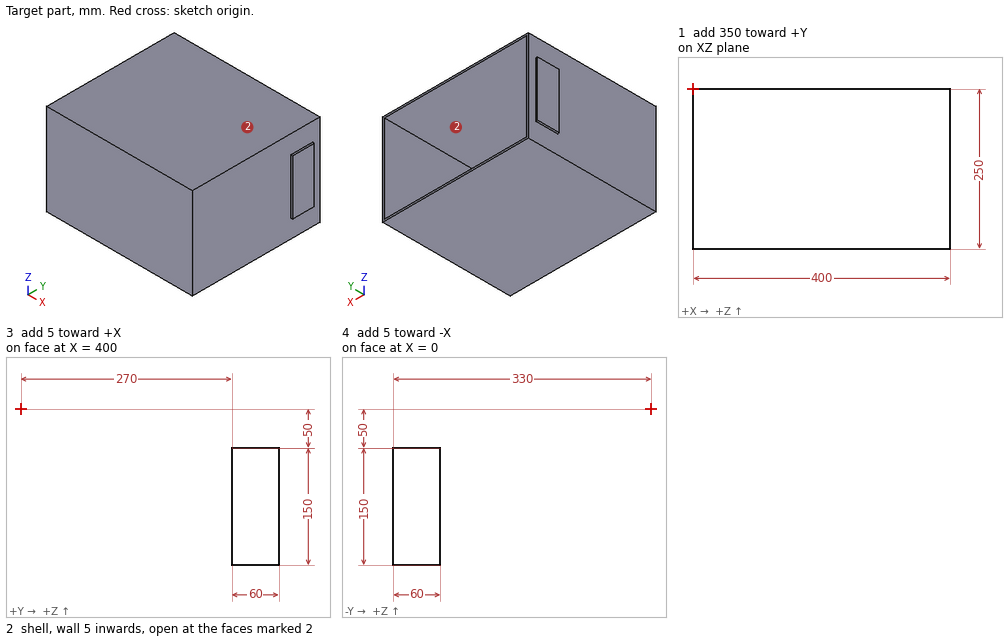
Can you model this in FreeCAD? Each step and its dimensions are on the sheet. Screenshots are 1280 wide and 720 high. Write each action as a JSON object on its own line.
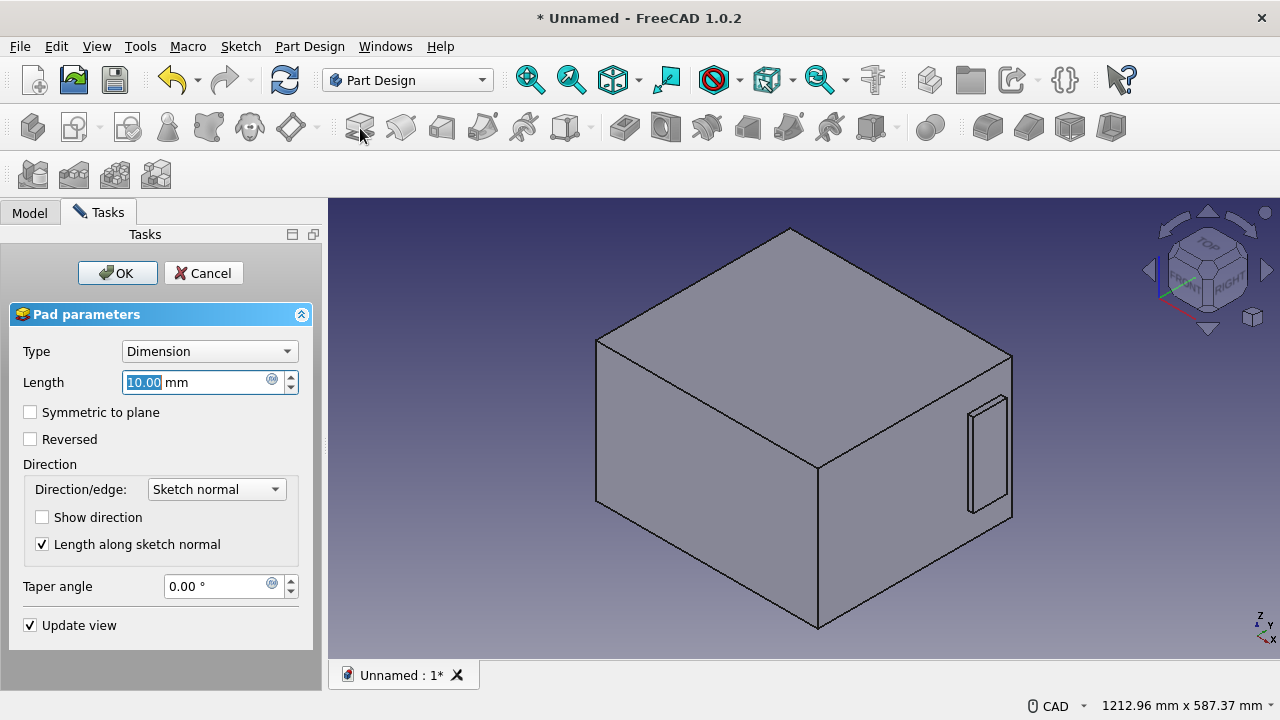
{"action": "type", "text": "5"}
{"action": "key", "text": "Tab"}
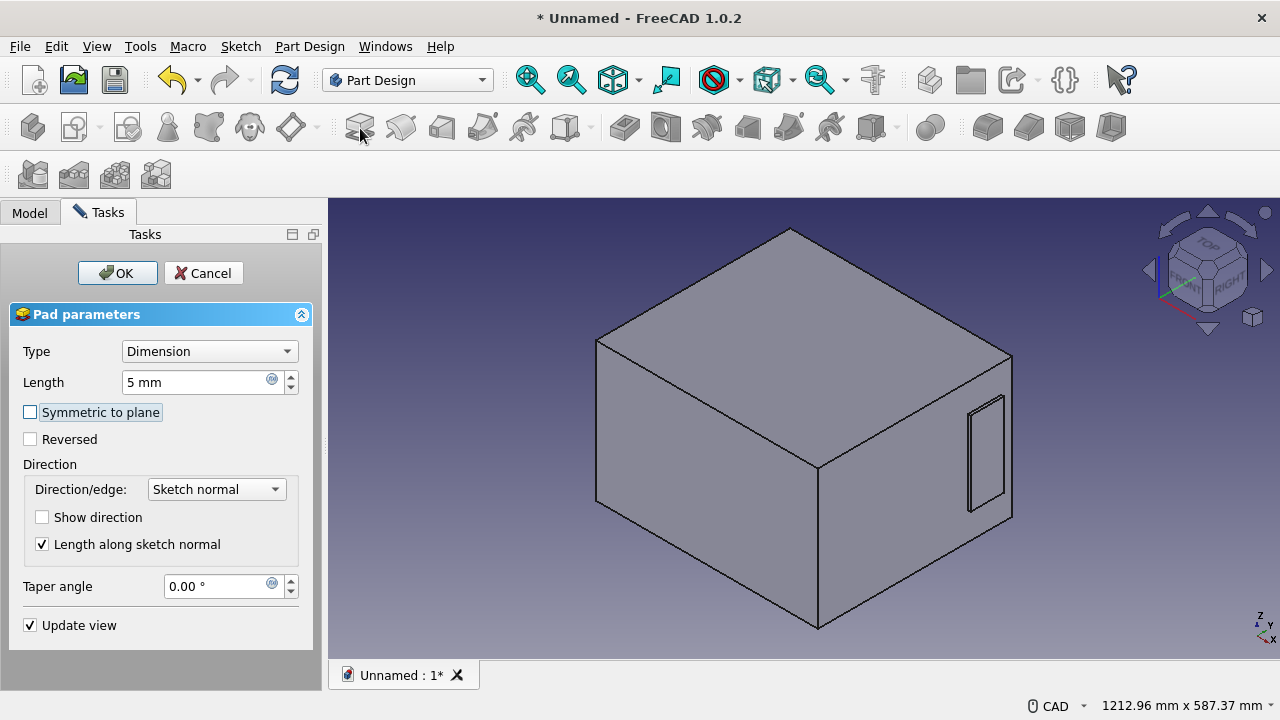
{"action": "left_click", "coordinate": [118, 273]}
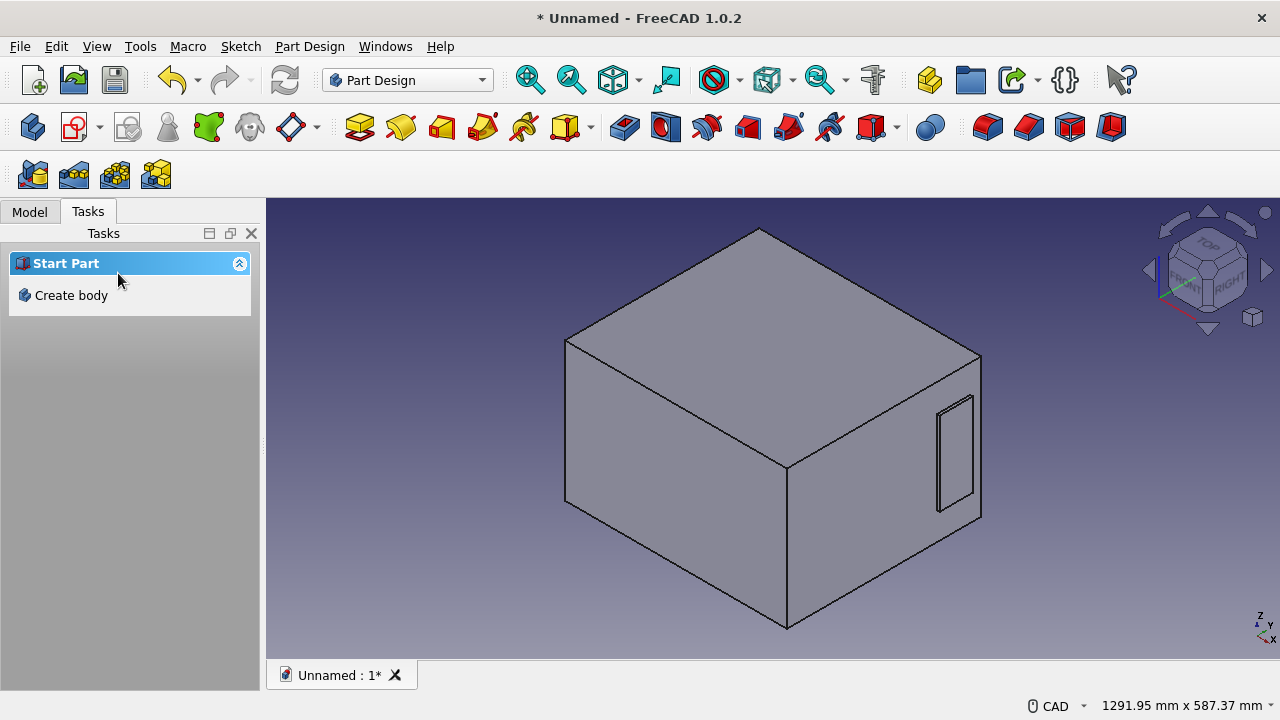
{"action": "key", "text": "6"}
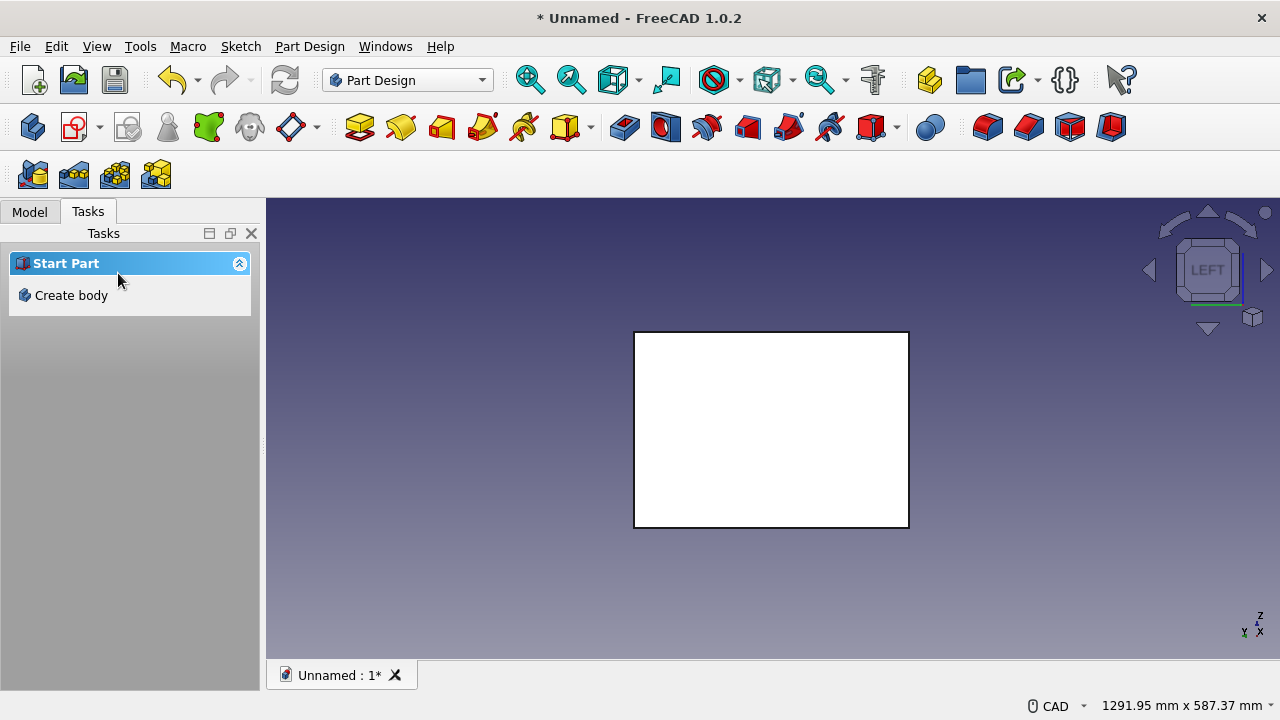
{"action": "left_click", "coordinate": [531, 80]}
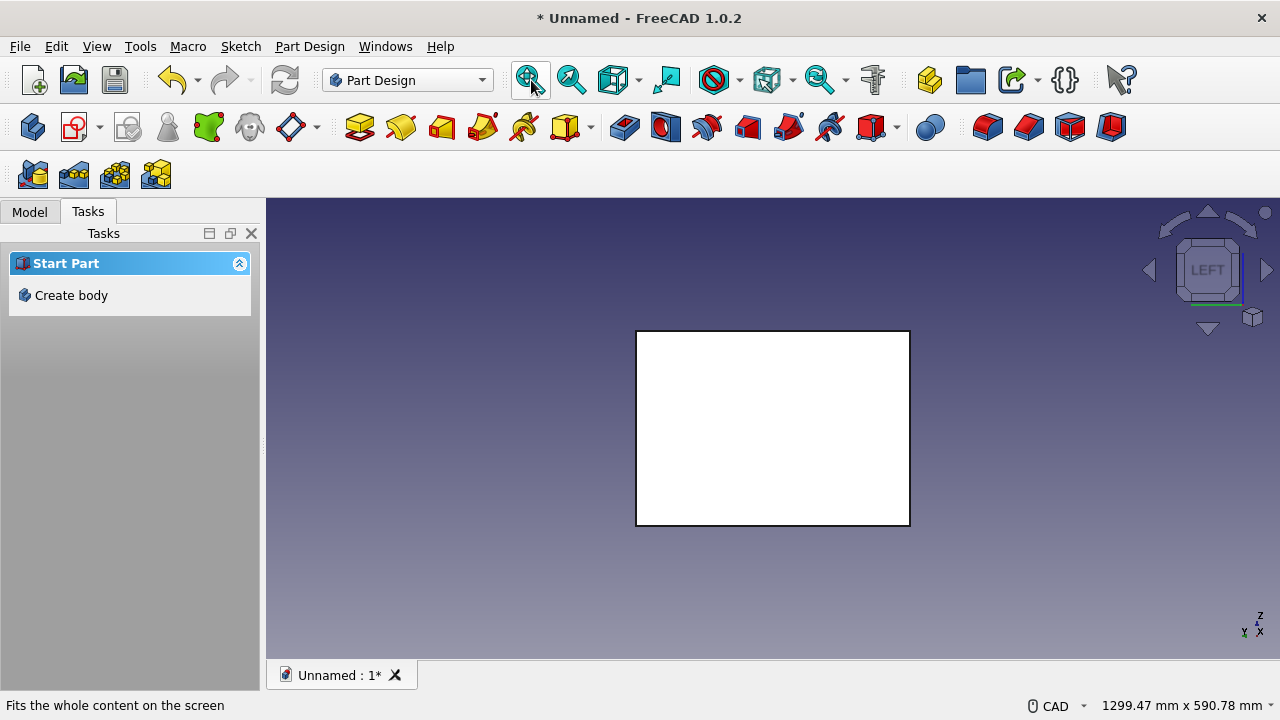
{"action": "left_click", "coordinate": [812, 427]}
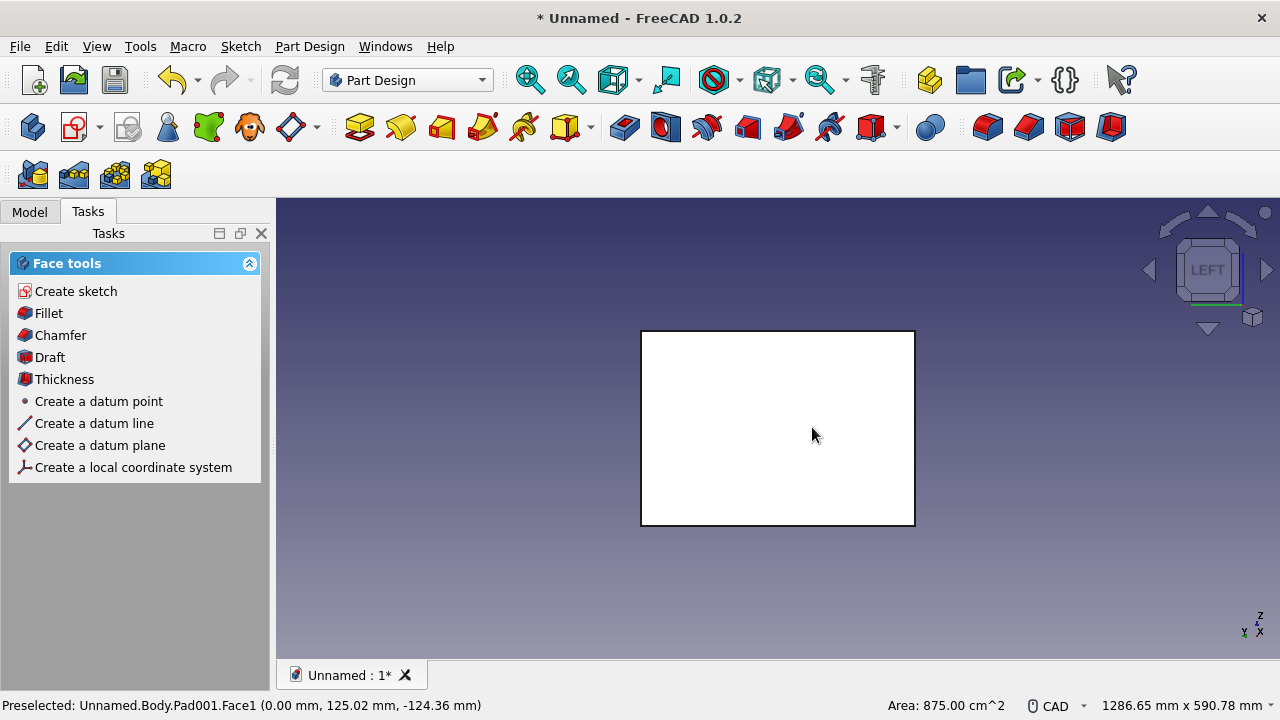
{"action": "left_click", "coordinate": [74, 128]}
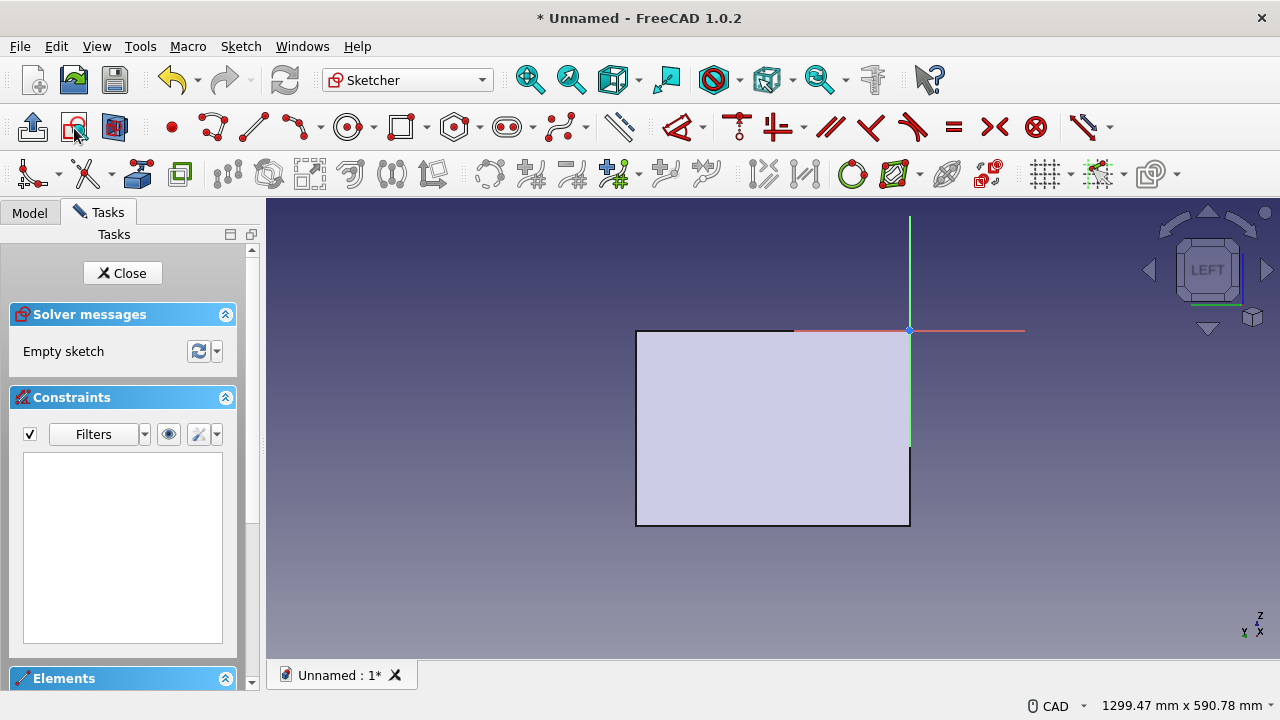
{"action": "scroll", "coordinate": [874, 385], "scroll_direction": "up", "scroll_amount": 3}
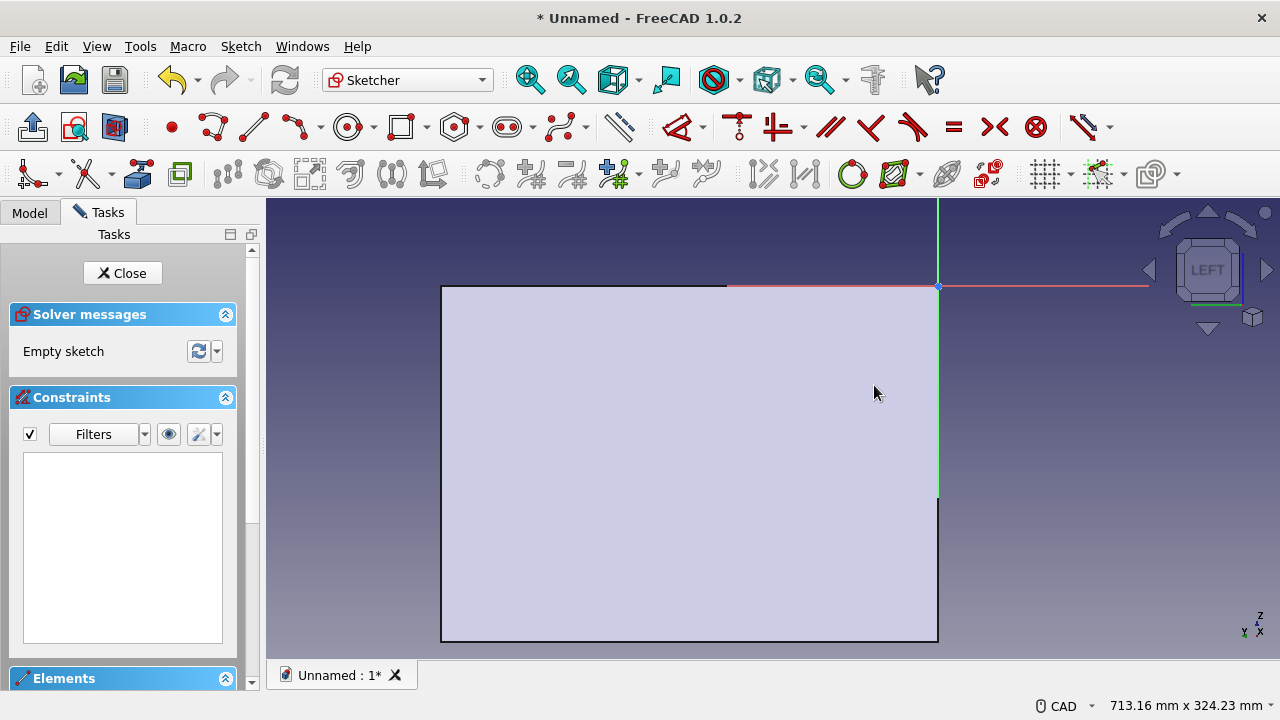
{"action": "key", "text": "g r"}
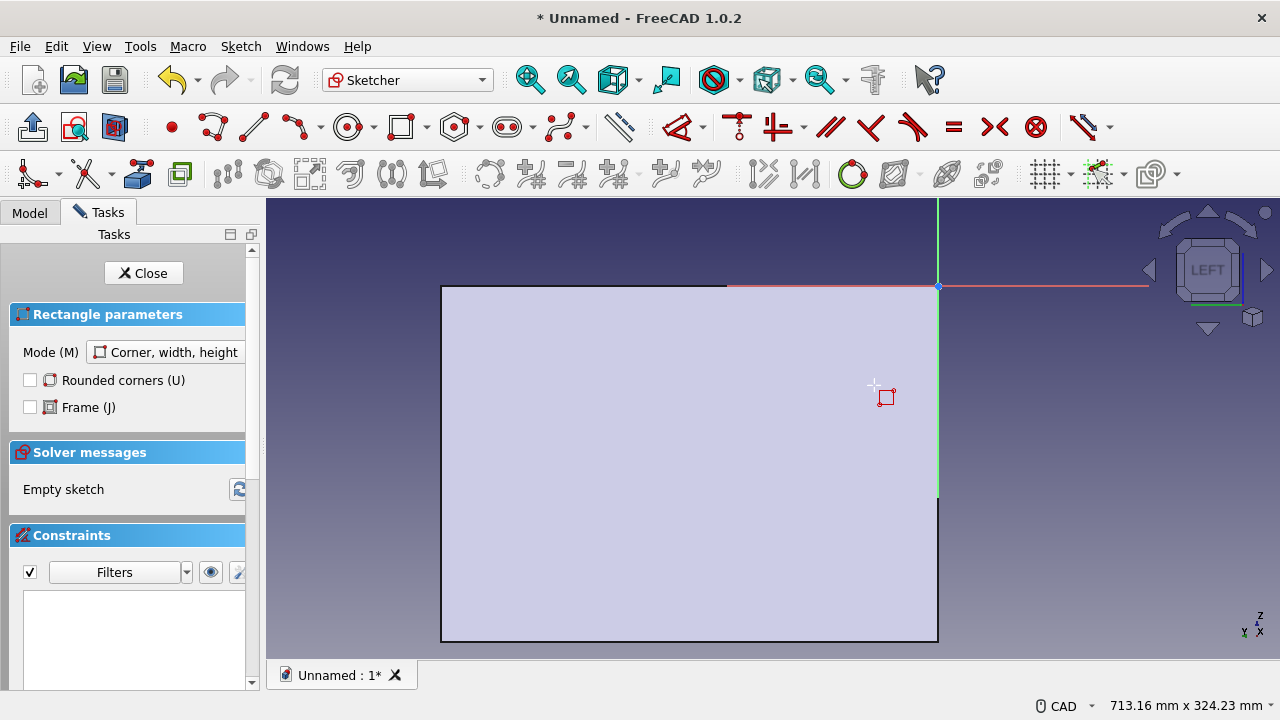
{"action": "left_click", "coordinate": [469, 357]}
{"action": "mouse_move", "coordinate": [554, 571]}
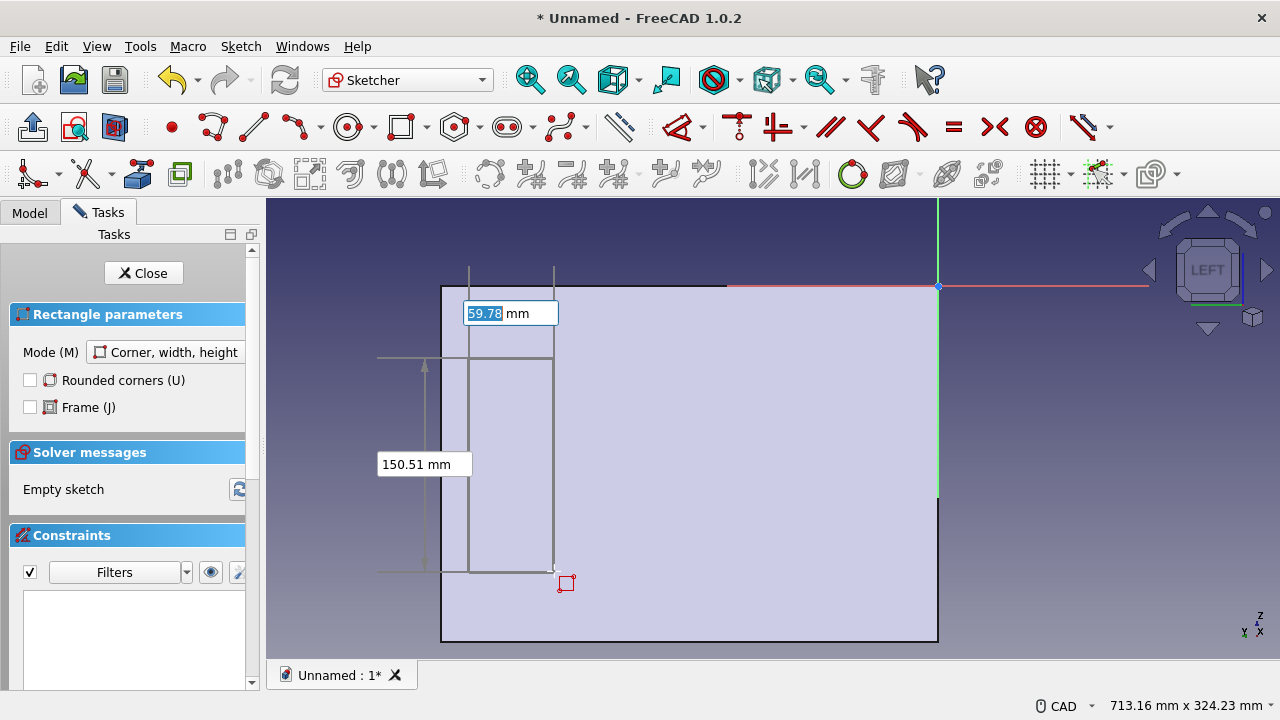
{"action": "type", "text": "60"}
{"action": "key", "text": "Tab"}
{"action": "type", "text": "150"}
{"action": "key", "text": "Return"}
{"action": "key", "text": "Escape"}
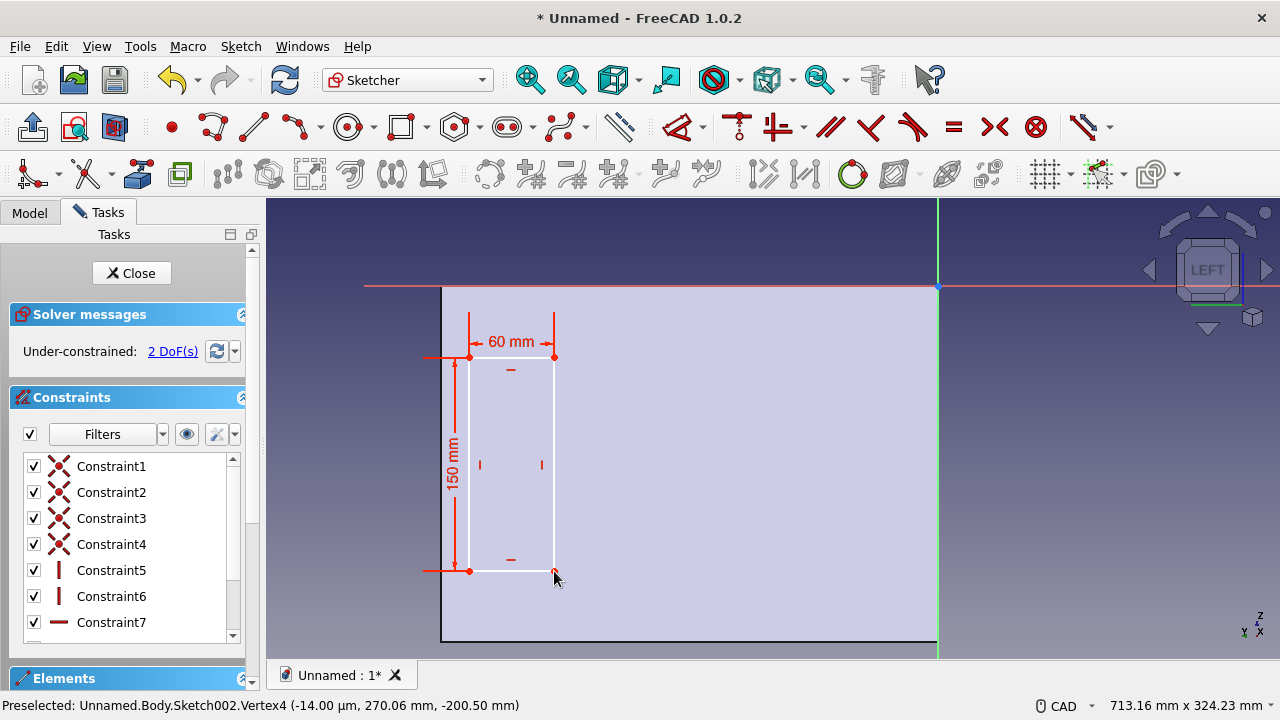
{"action": "left_click", "coordinate": [676, 128]}